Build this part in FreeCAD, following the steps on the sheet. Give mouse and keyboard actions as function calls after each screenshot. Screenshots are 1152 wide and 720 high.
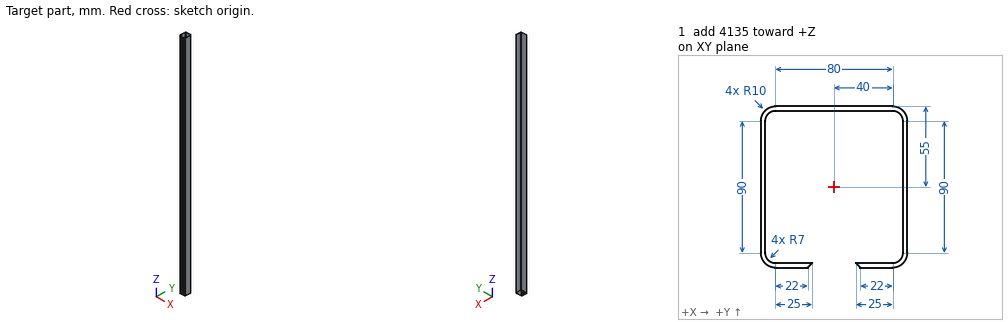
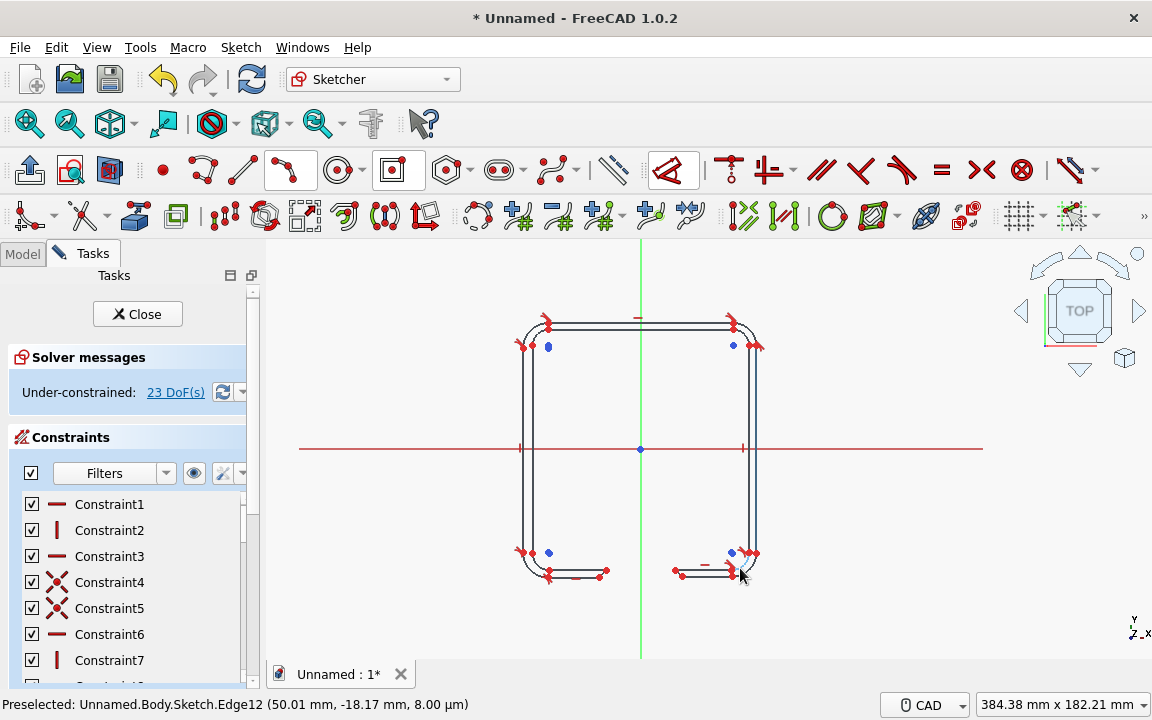
scroll(754, 335, up, 4)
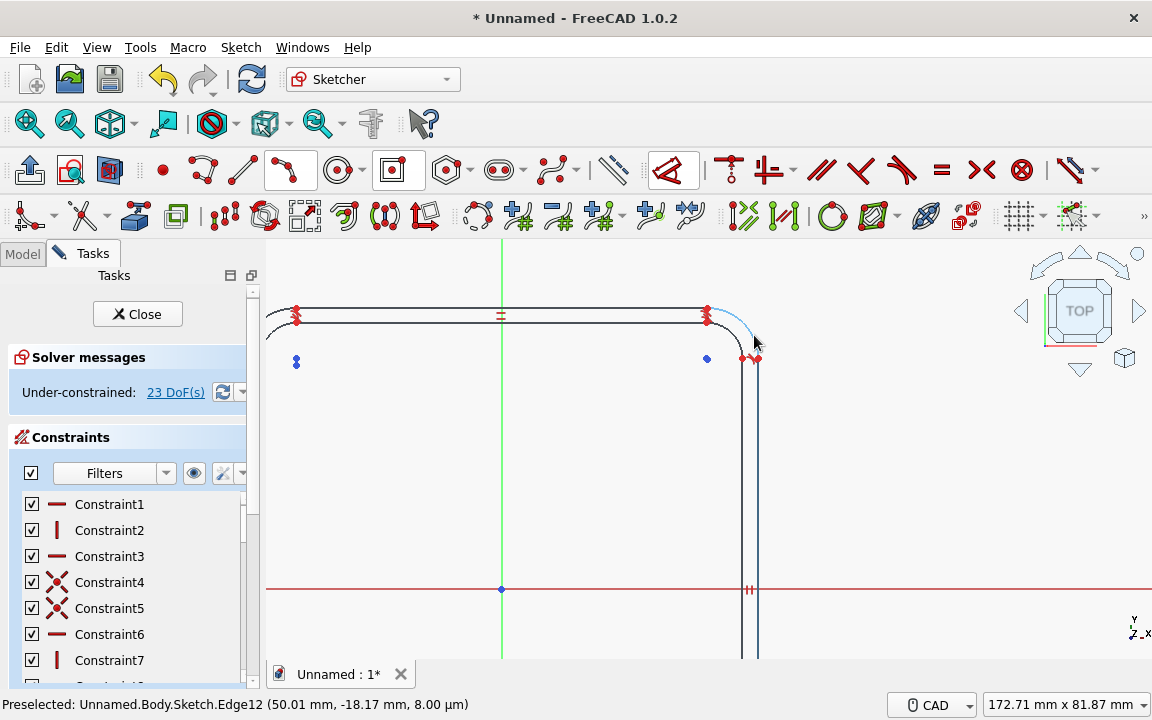
click(753, 336)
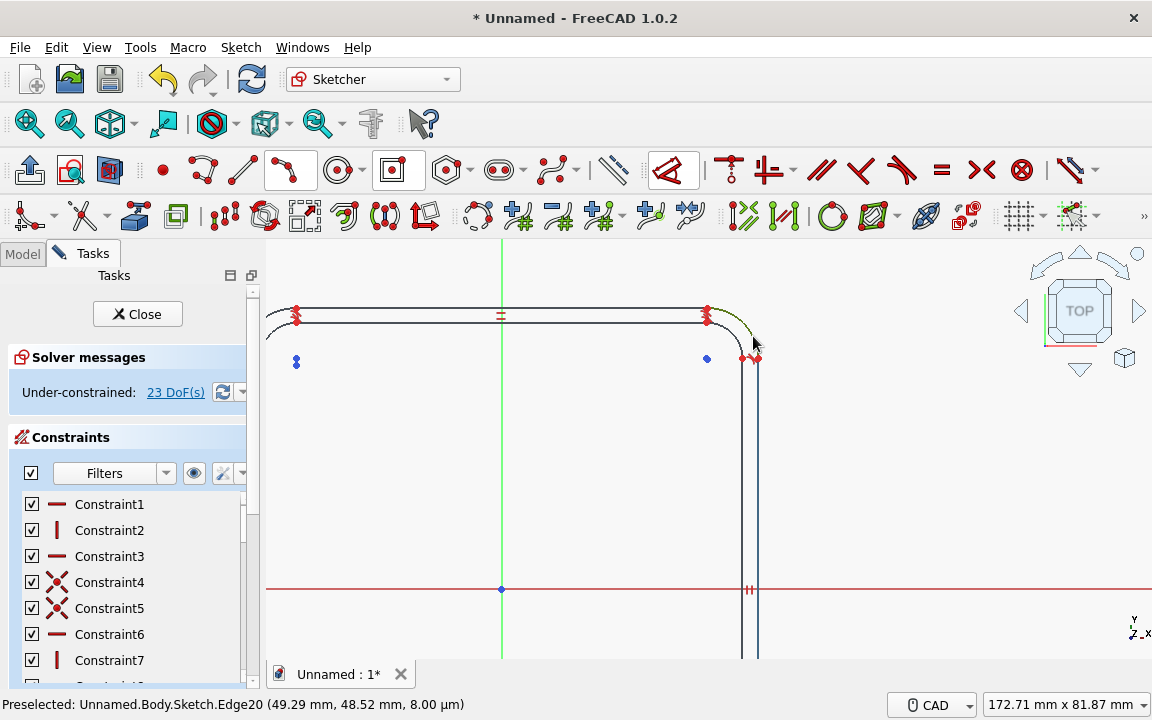
click(902, 170)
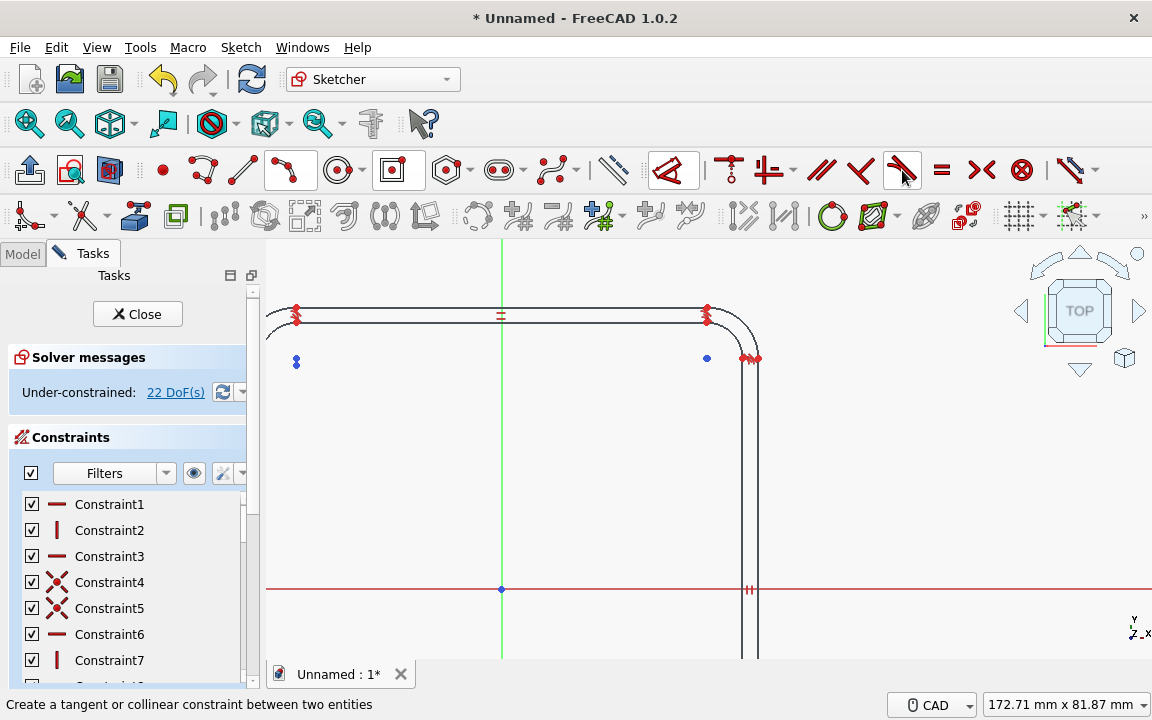
scroll(754, 335, down, 4)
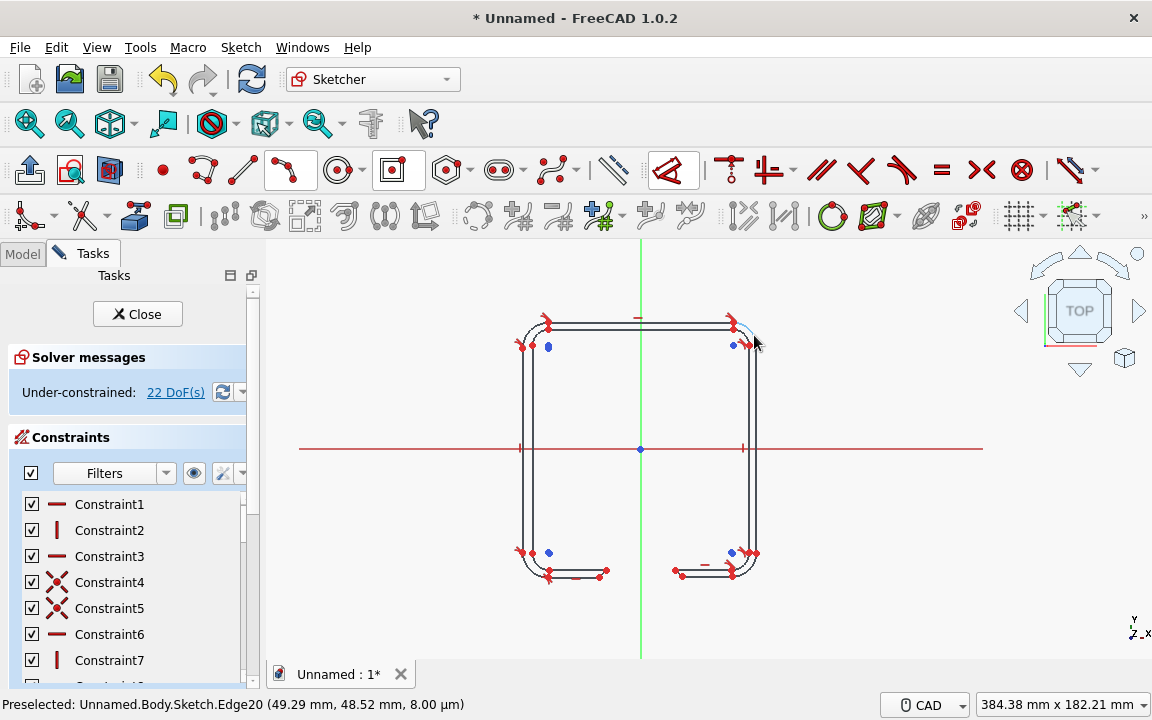
scroll(526, 564, up, 3)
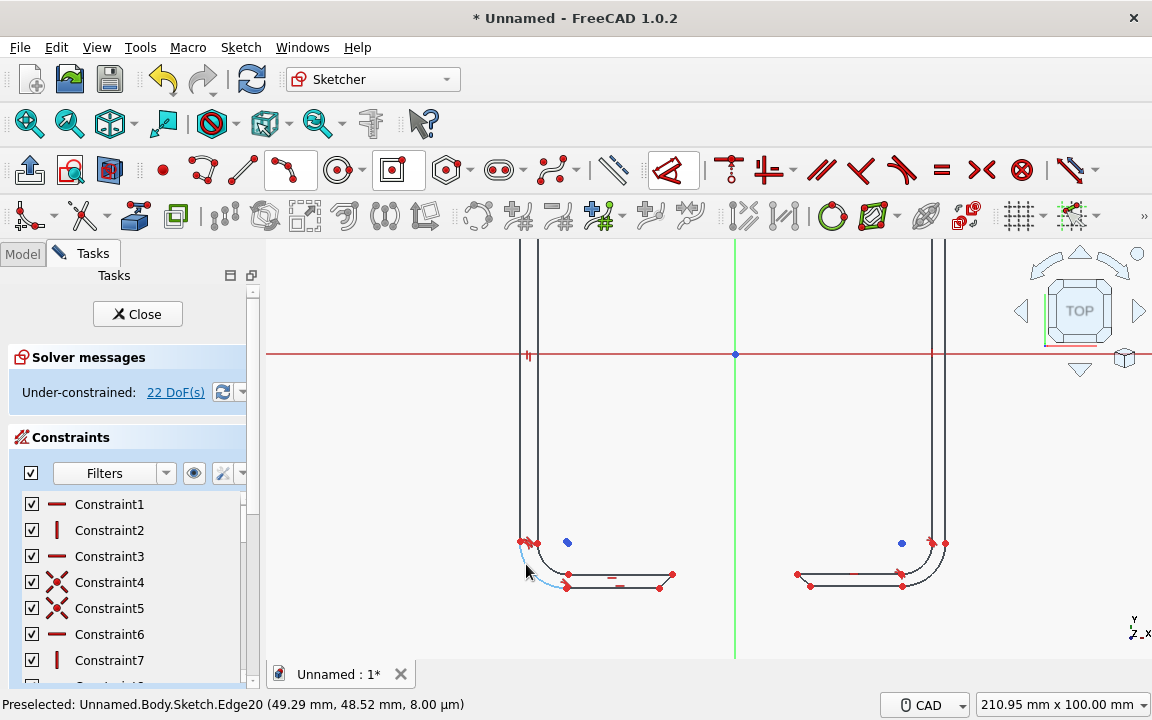
click(525, 563)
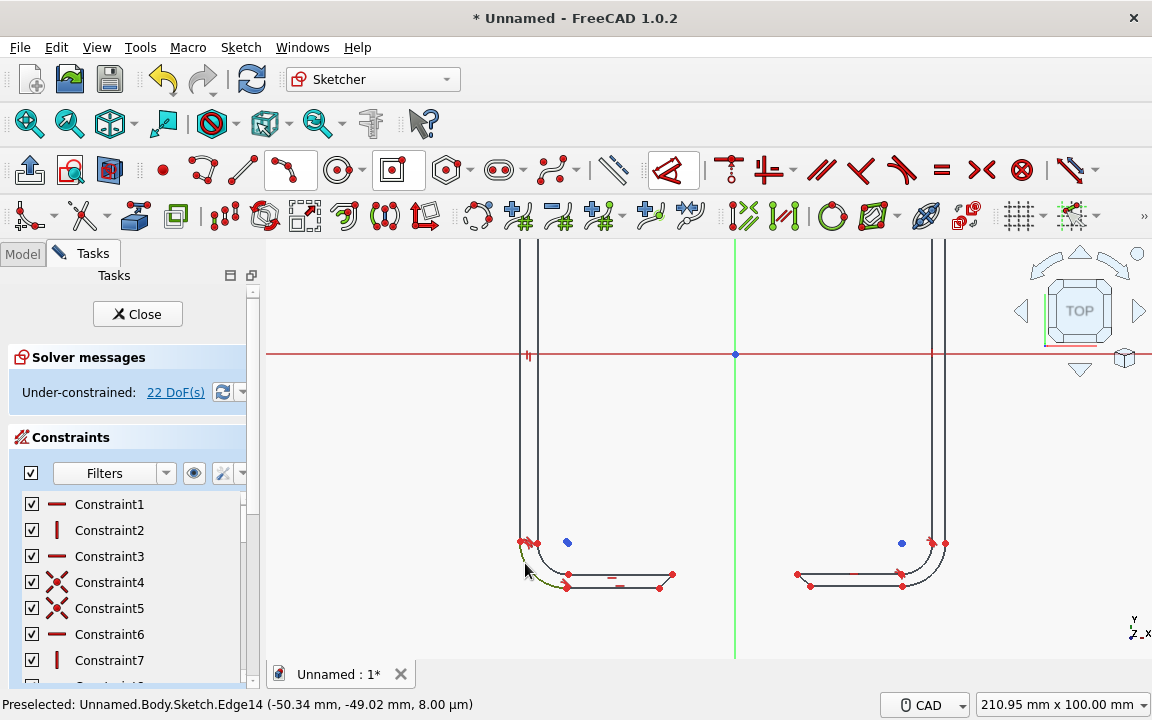
click(541, 558)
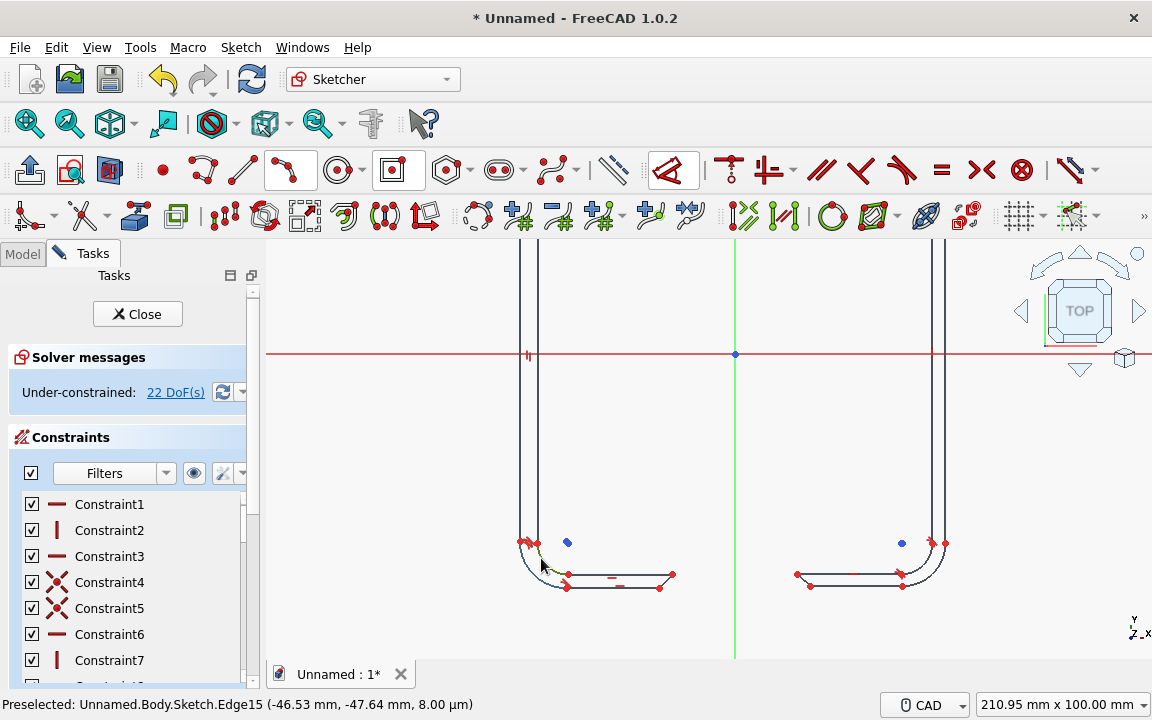
click(730, 170)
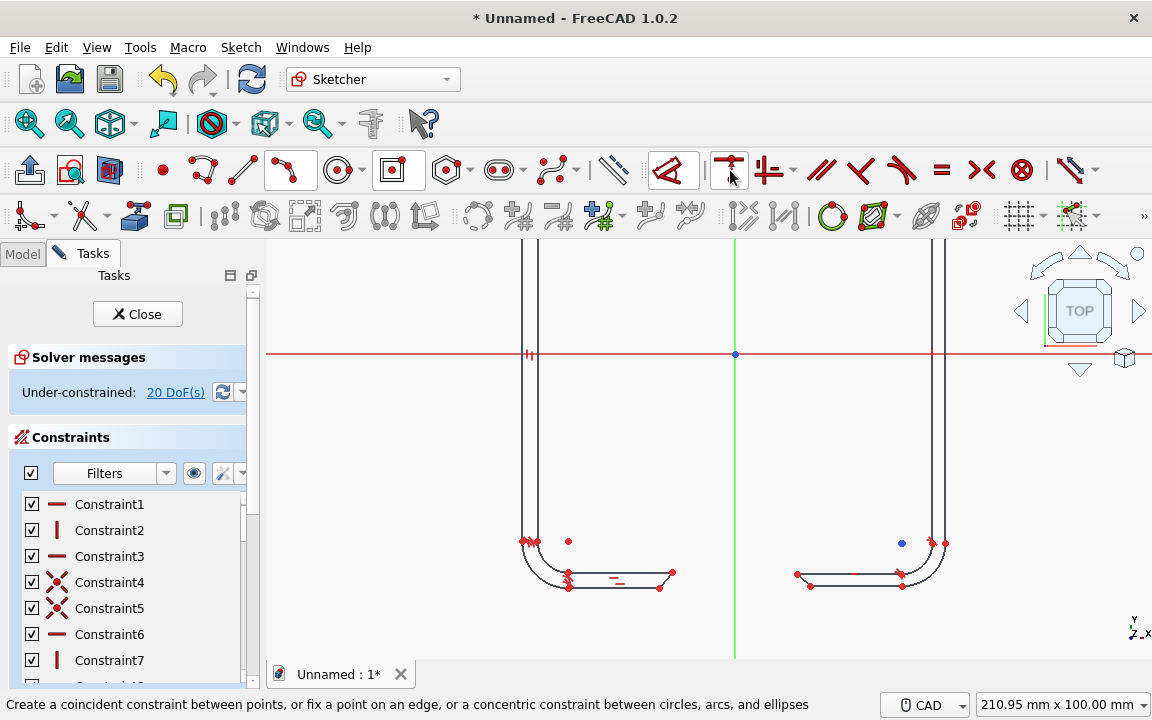
scroll(525, 564, down, 3)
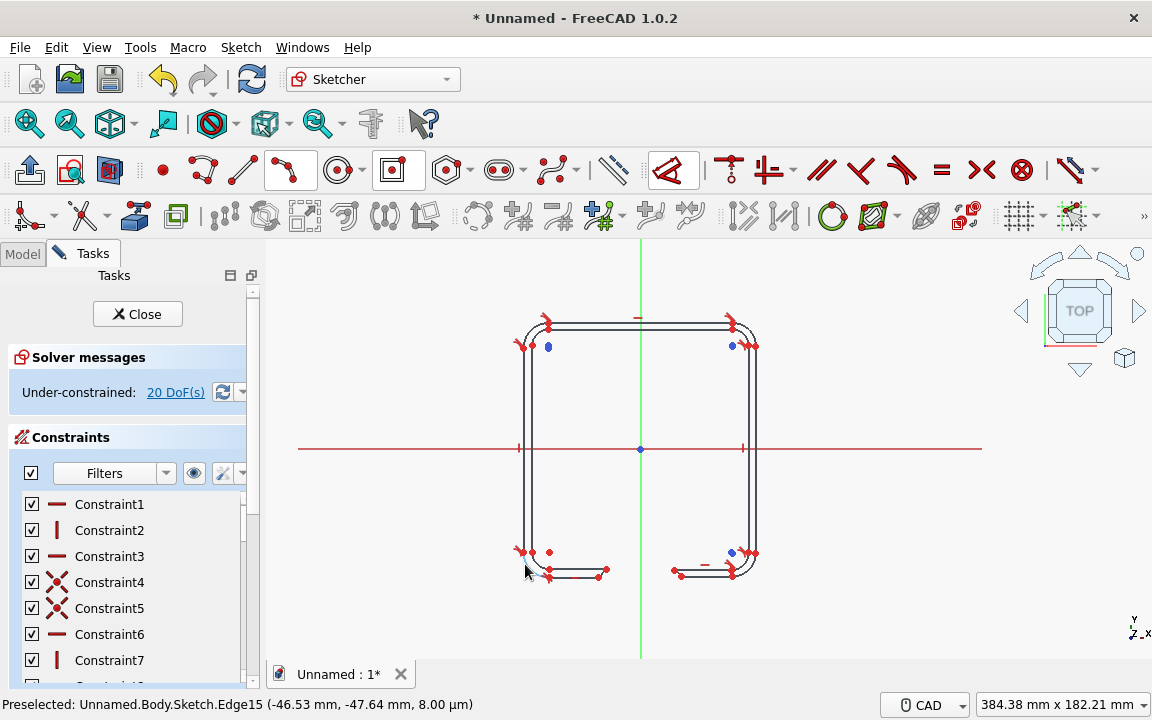
scroll(537, 326, up, 4)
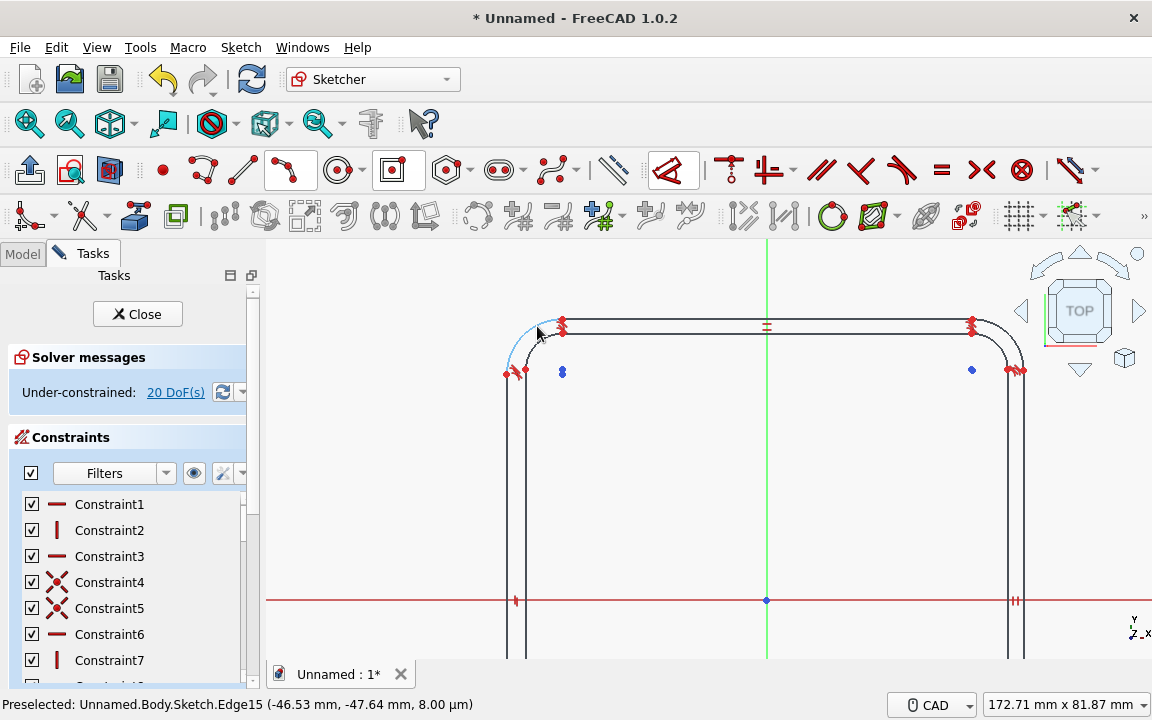
click(537, 325)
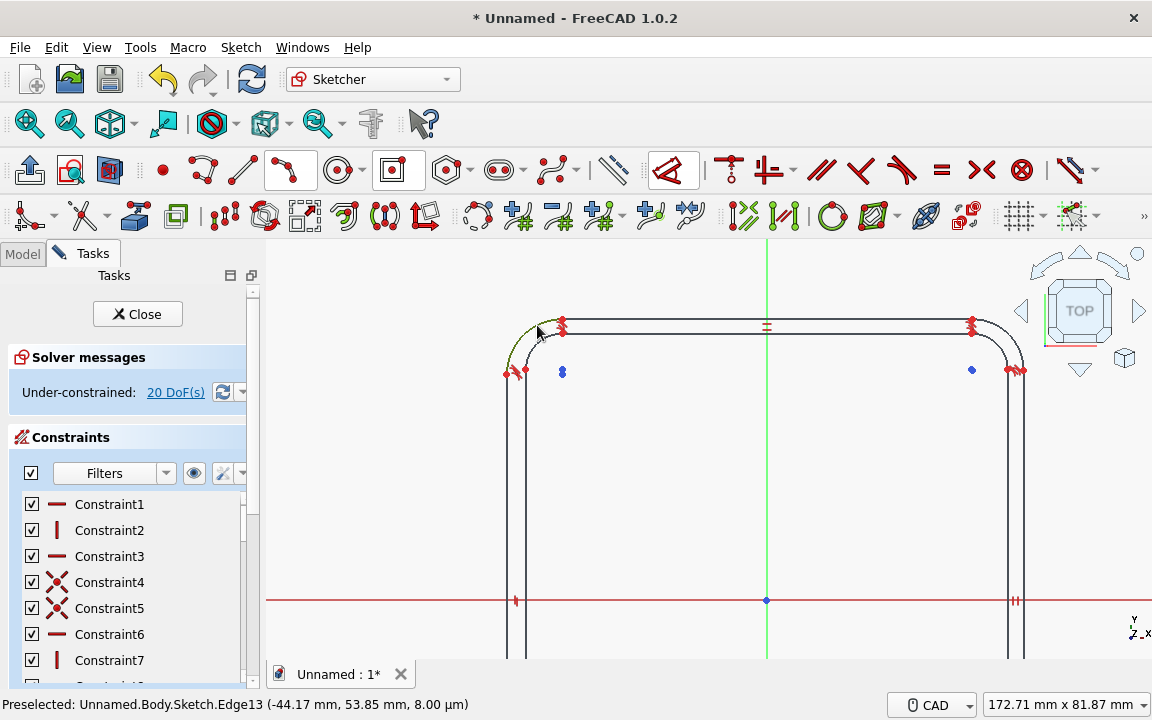
click(546, 338)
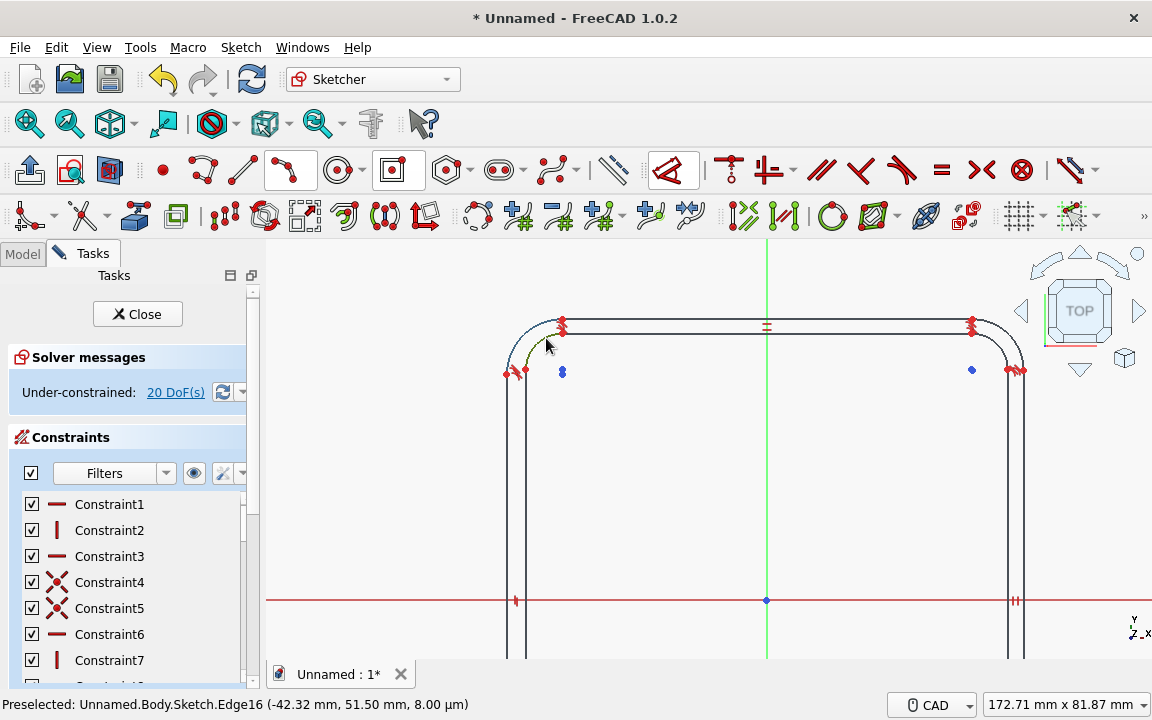
click(730, 170)